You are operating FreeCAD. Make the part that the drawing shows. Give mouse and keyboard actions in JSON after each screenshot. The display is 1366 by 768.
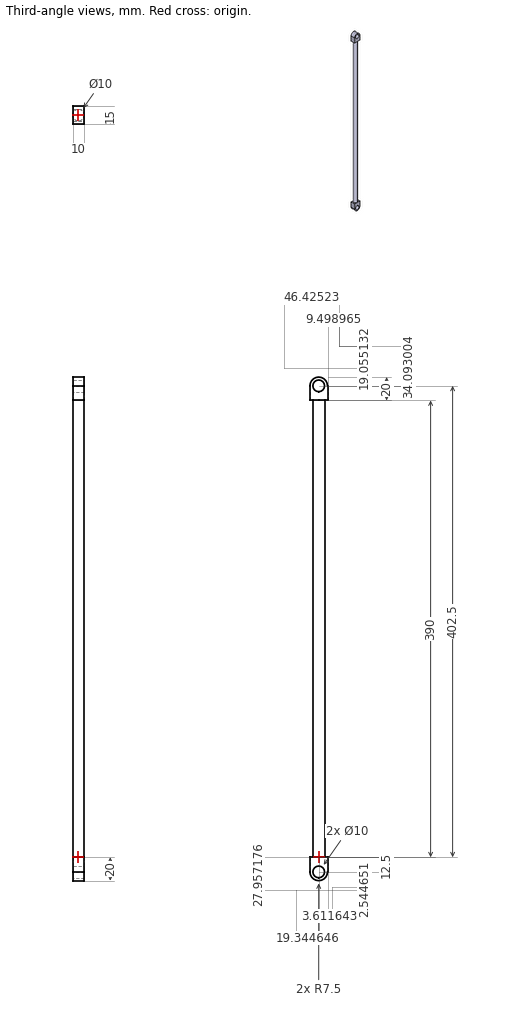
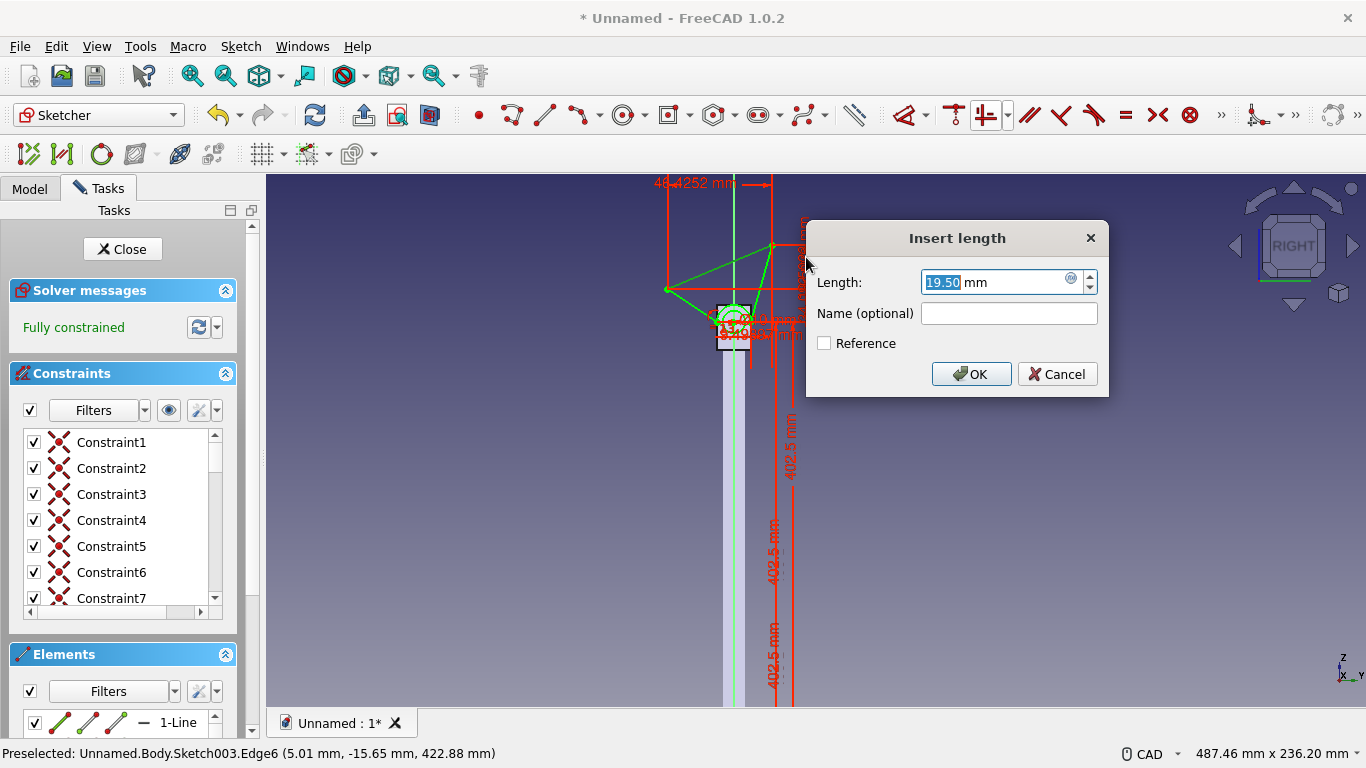
{"action": "type", "text": "19.055132"}
{"action": "key", "text": "Return"}
{"action": "key", "text": "Escape"}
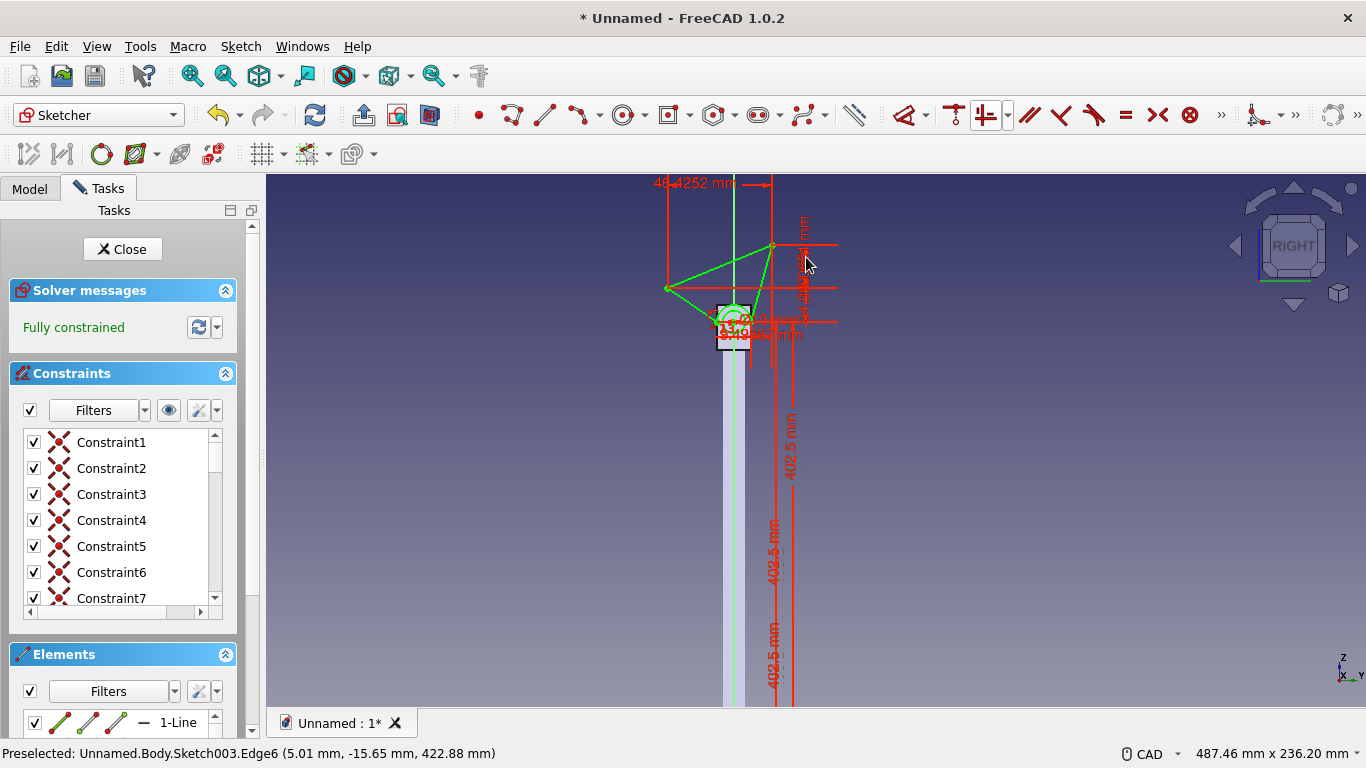
{"action": "left_click", "coordinate": [123, 249]}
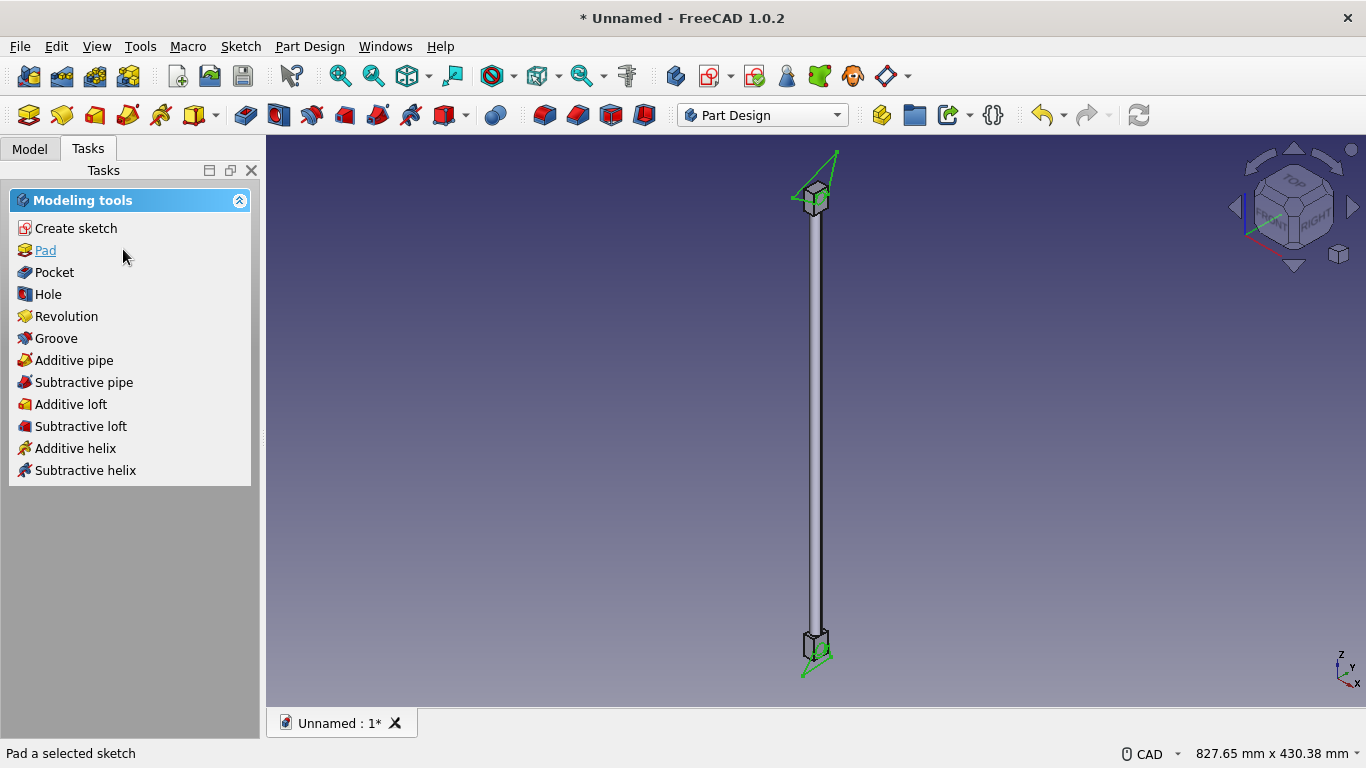
{"action": "left_click", "coordinate": [246, 116]}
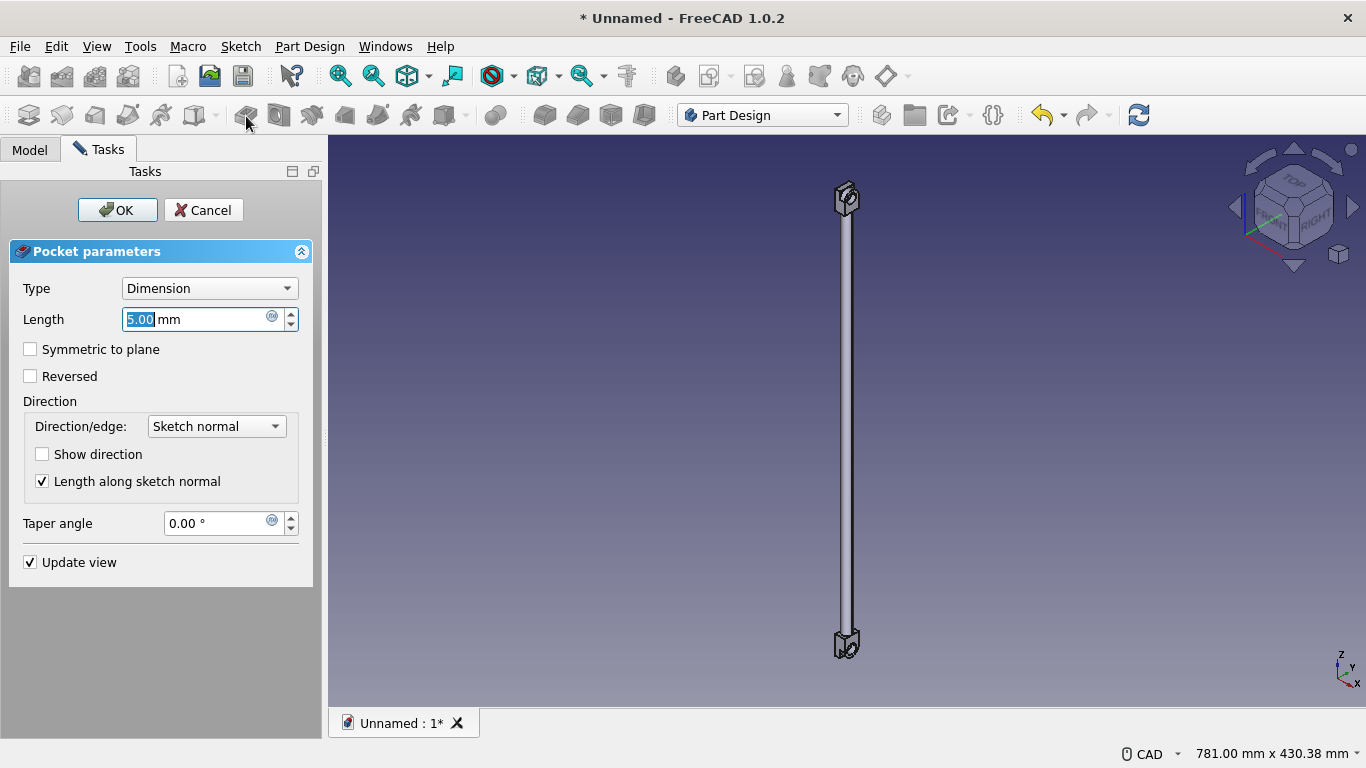
{"action": "left_click", "coordinate": [210, 288]}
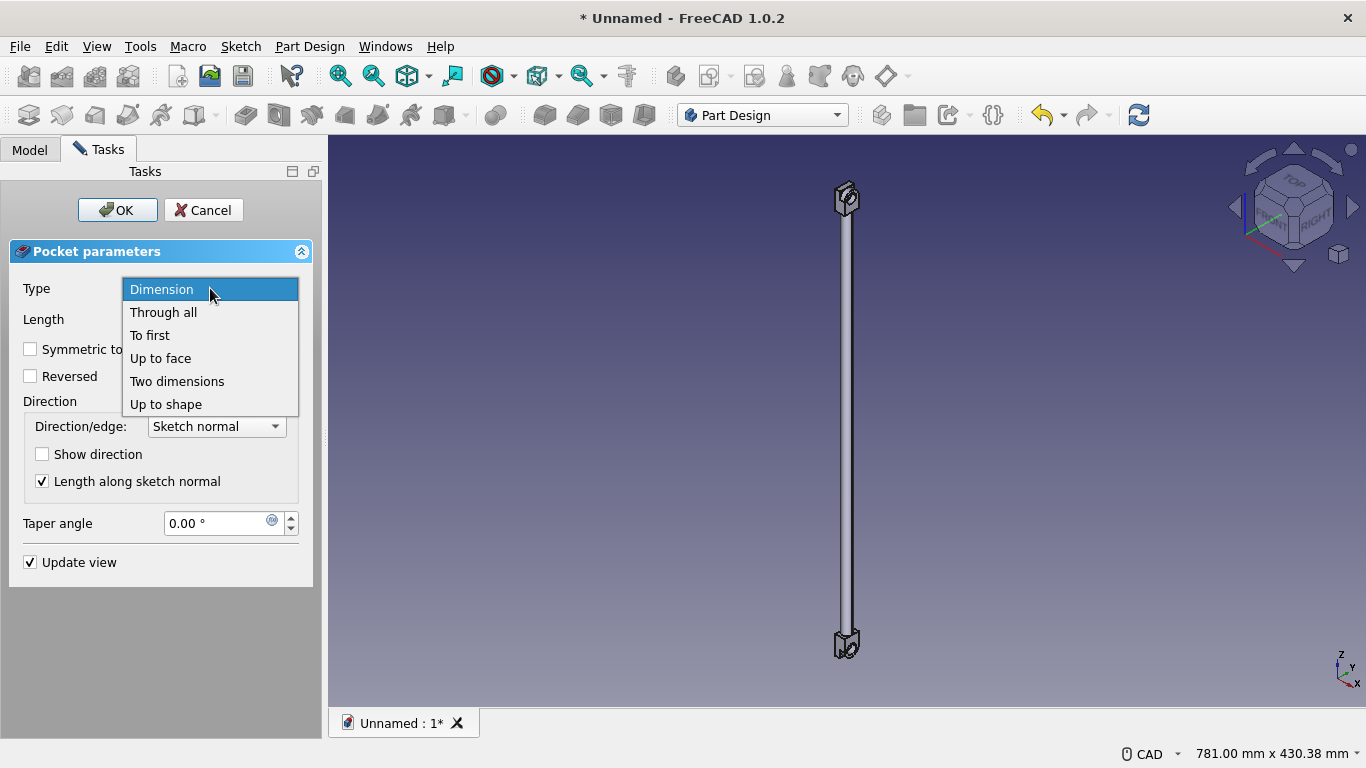
{"action": "left_click", "coordinate": [208, 312]}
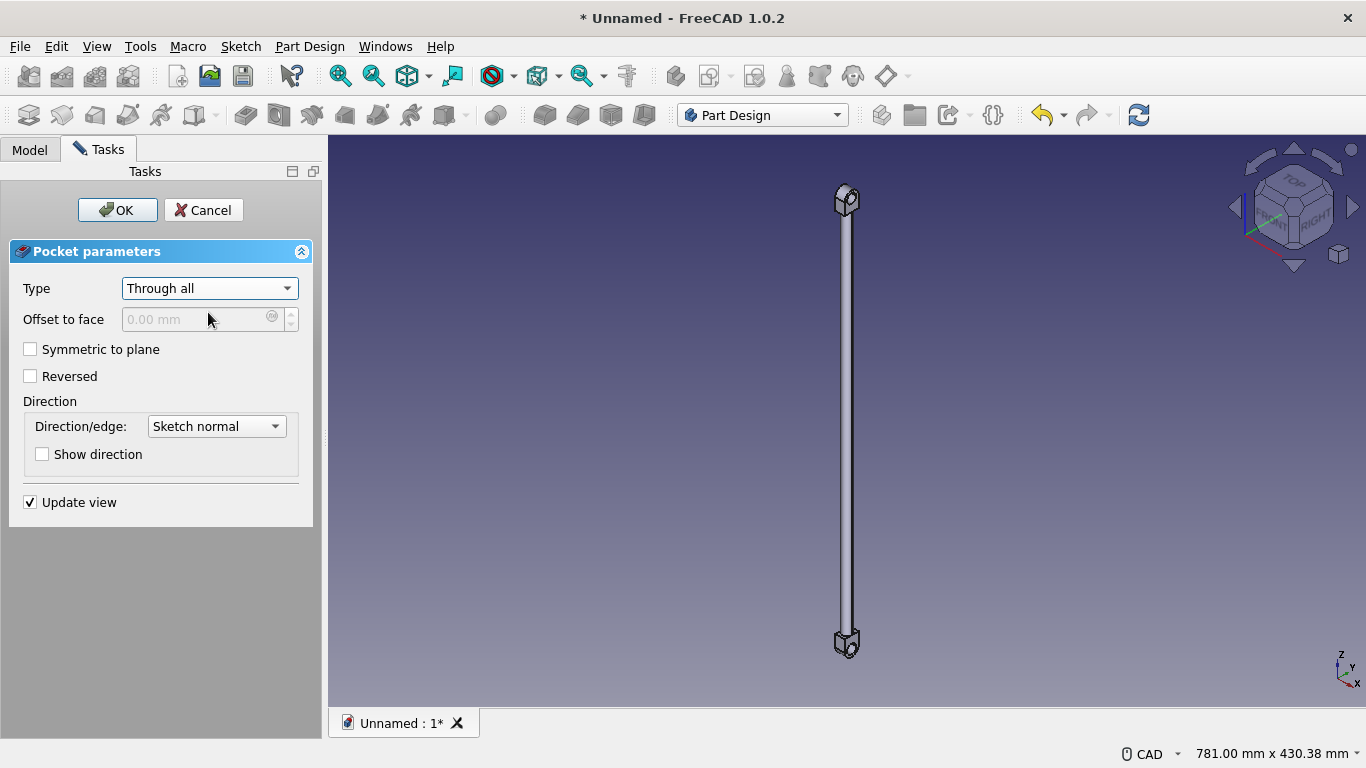
{"action": "left_click", "coordinate": [118, 210]}